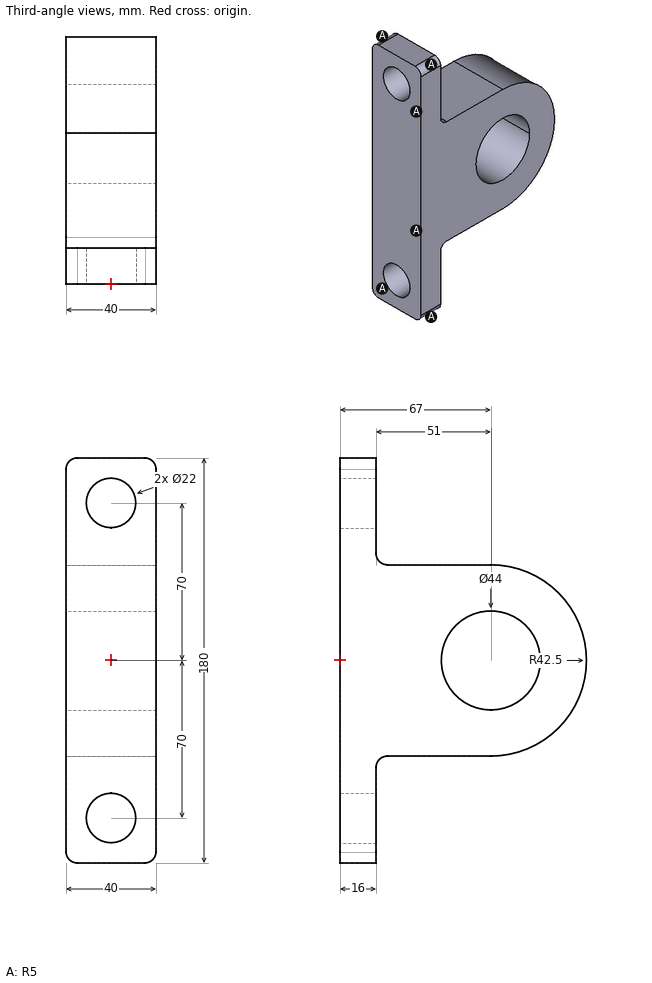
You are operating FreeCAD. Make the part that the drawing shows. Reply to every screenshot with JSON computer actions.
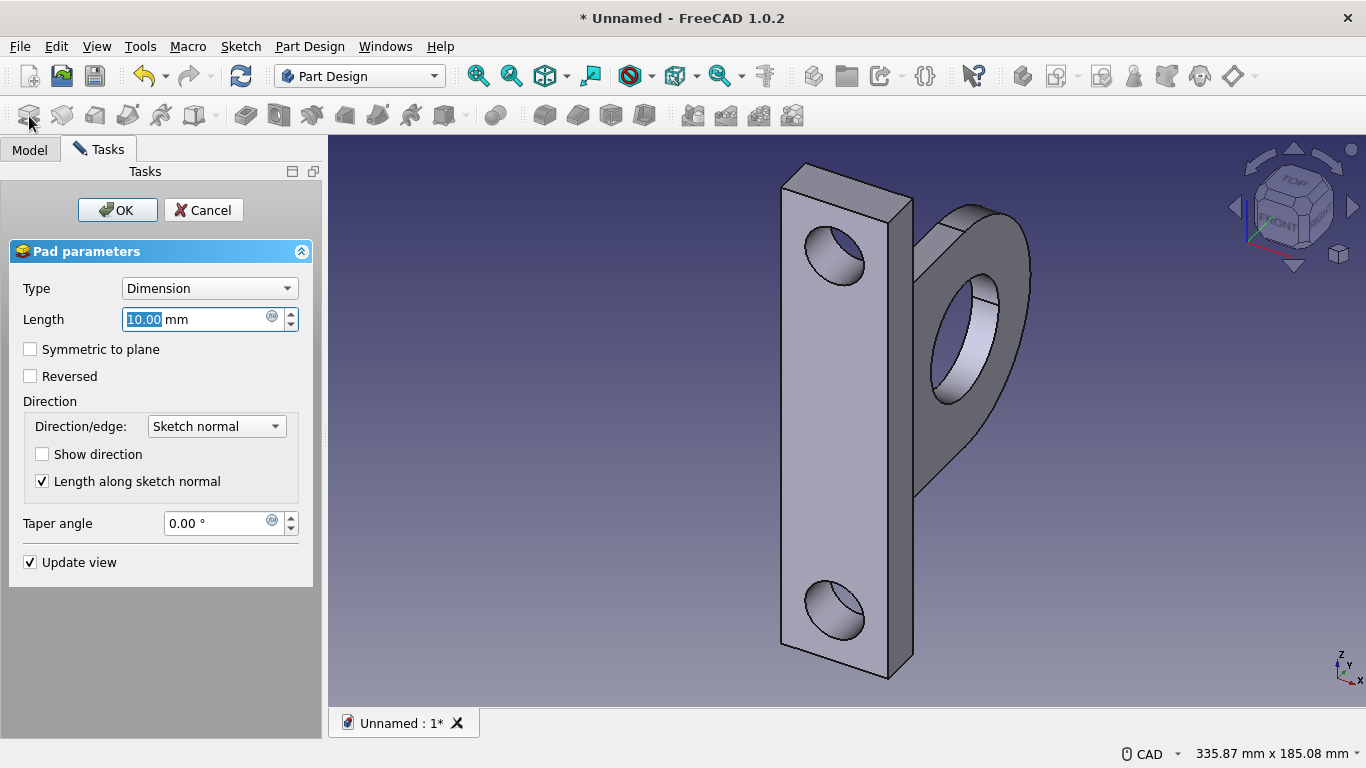
{"action": "type", "text": "40"}
{"action": "key", "text": "Tab"}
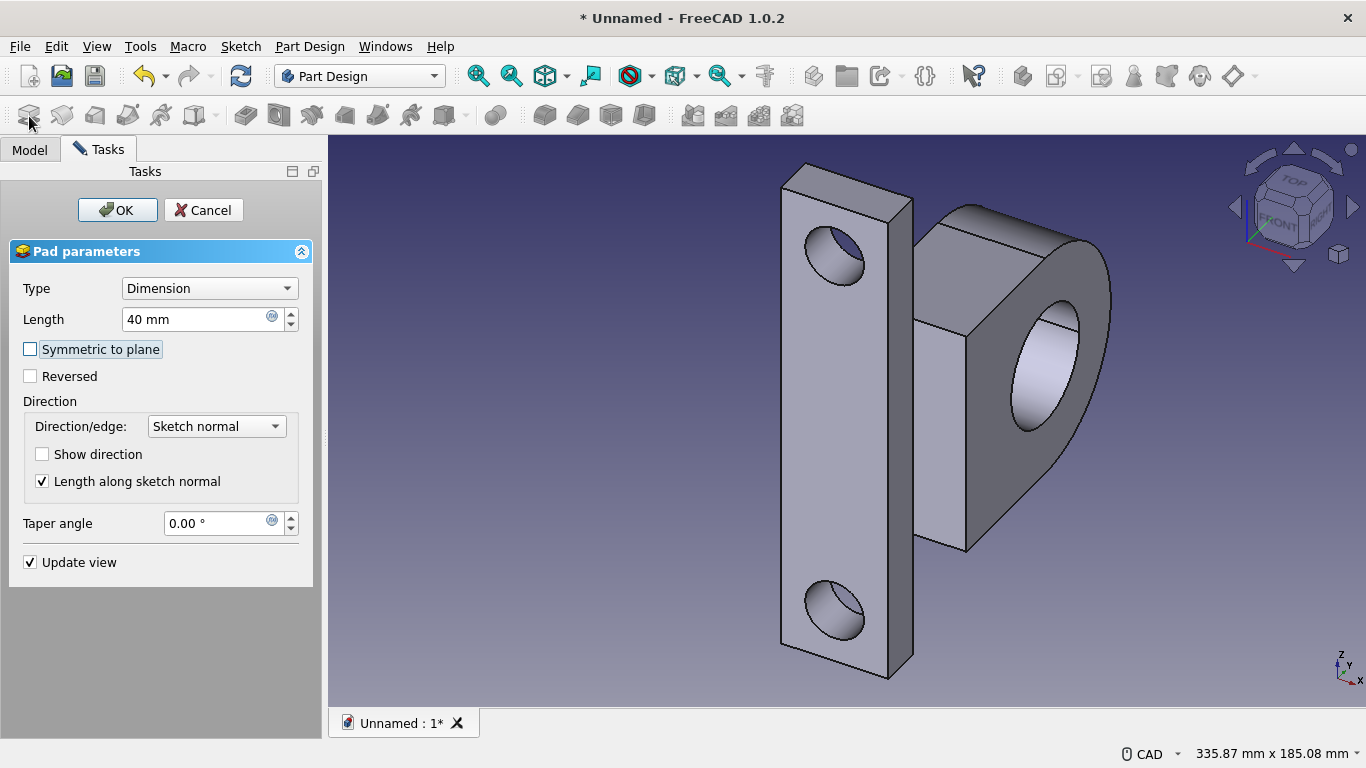
{"action": "left_click", "coordinate": [31, 349]}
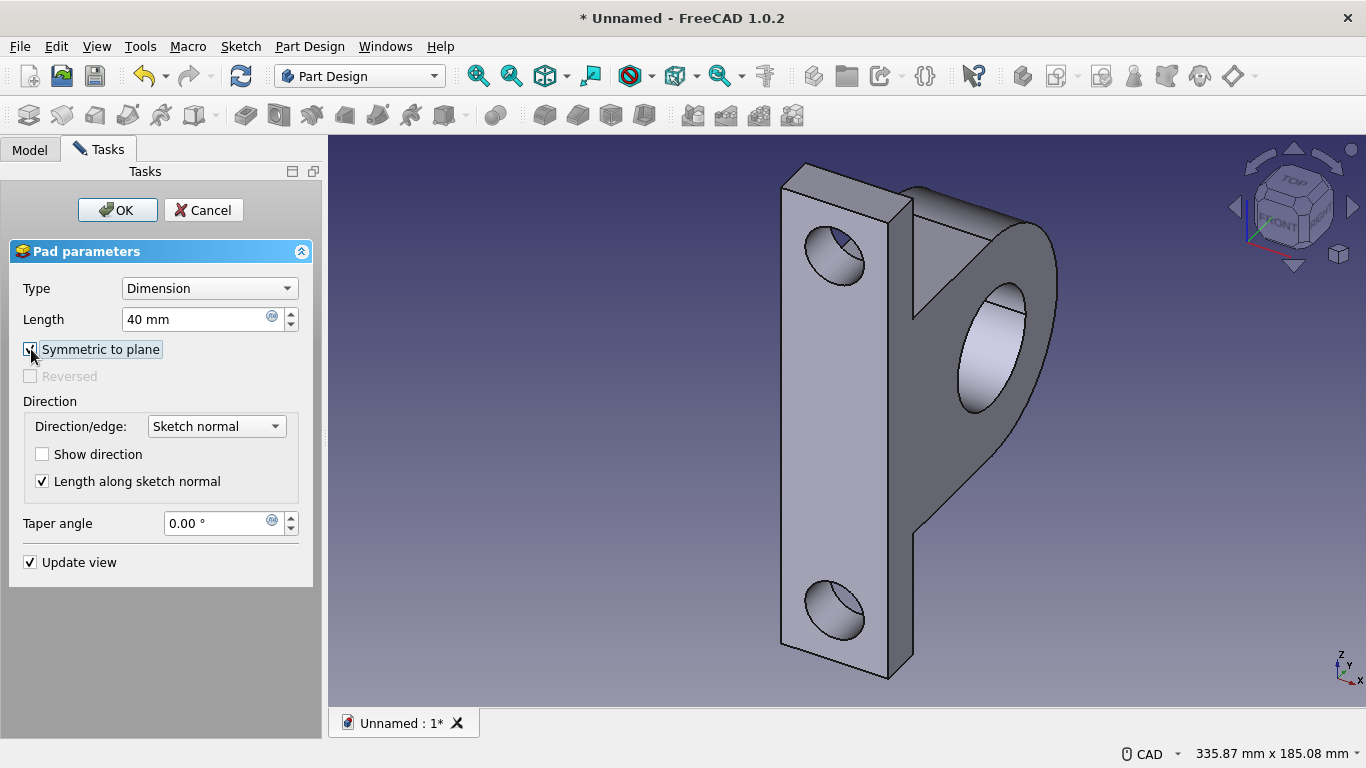
{"action": "left_click", "coordinate": [118, 210]}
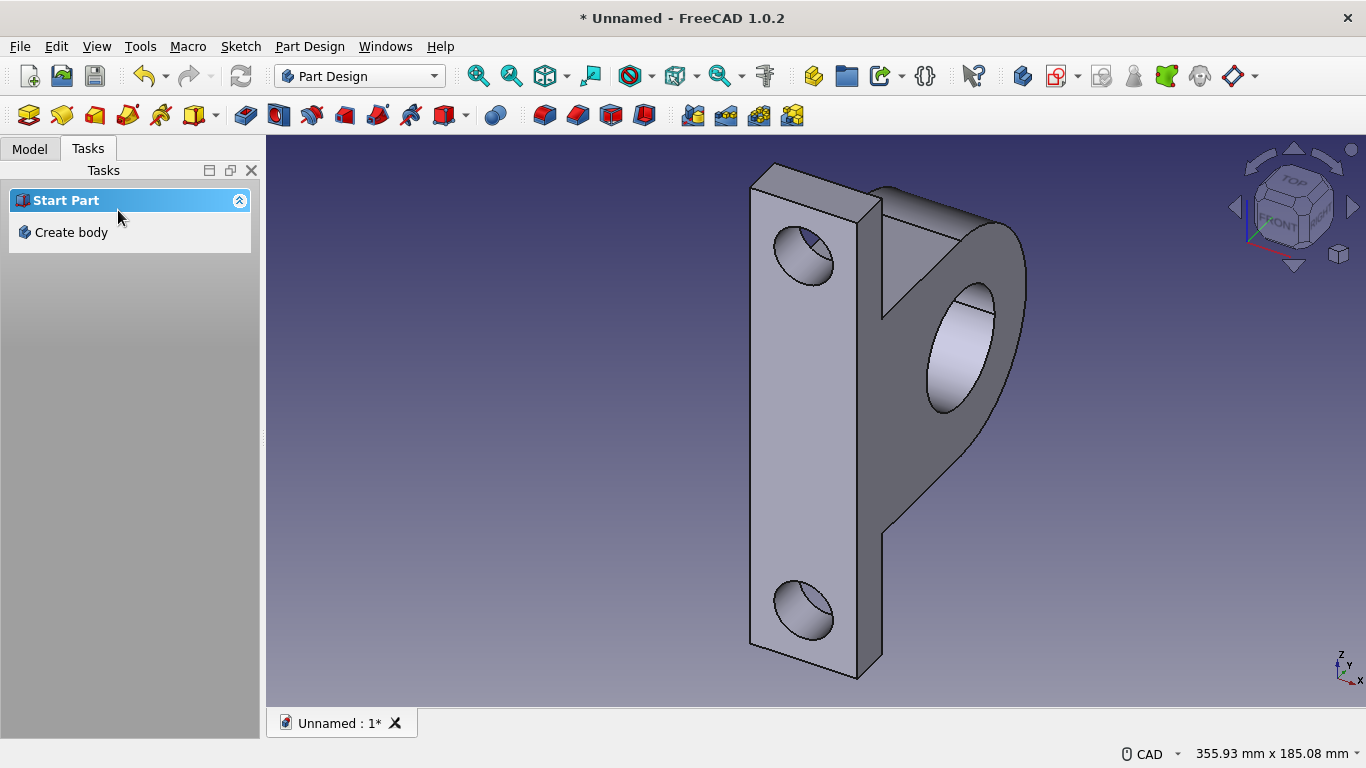
{"action": "key", "text": "v f"}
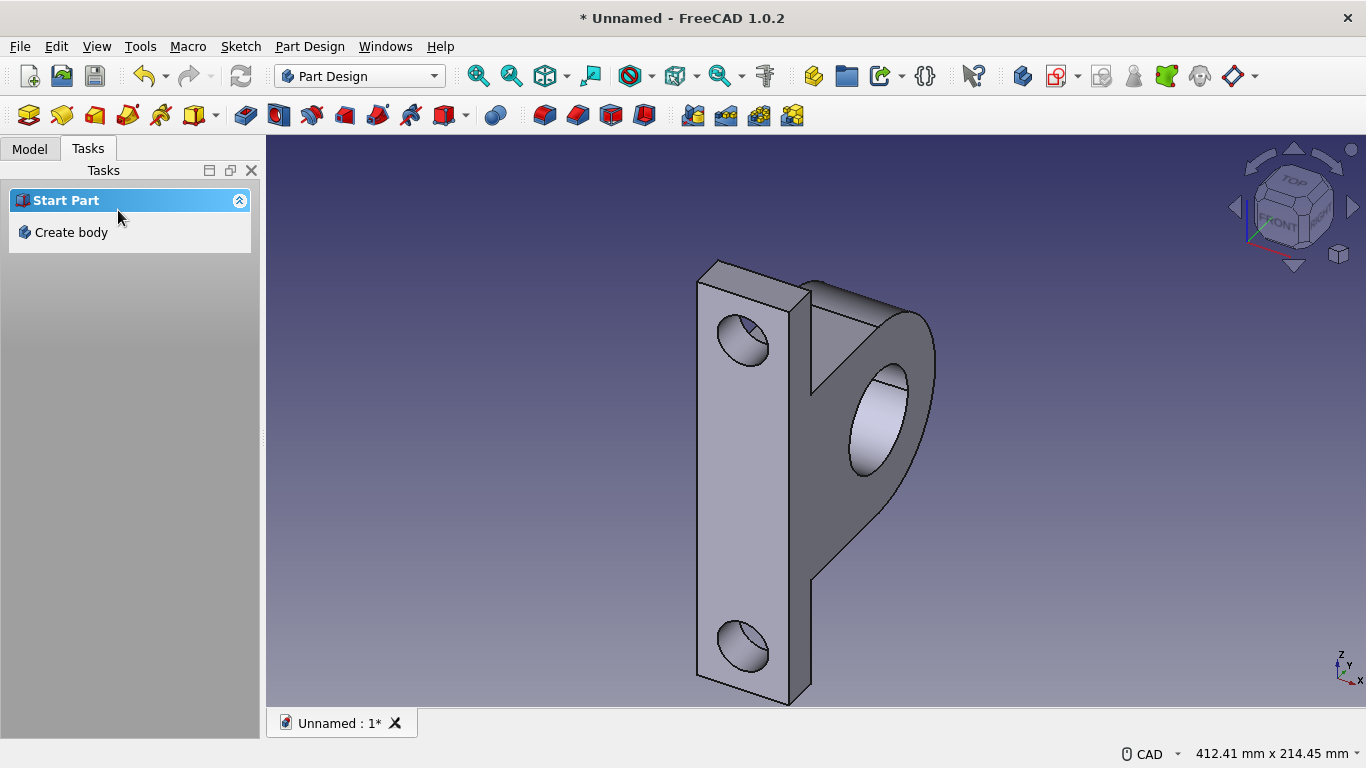
{"action": "left_click", "coordinate": [800, 301]}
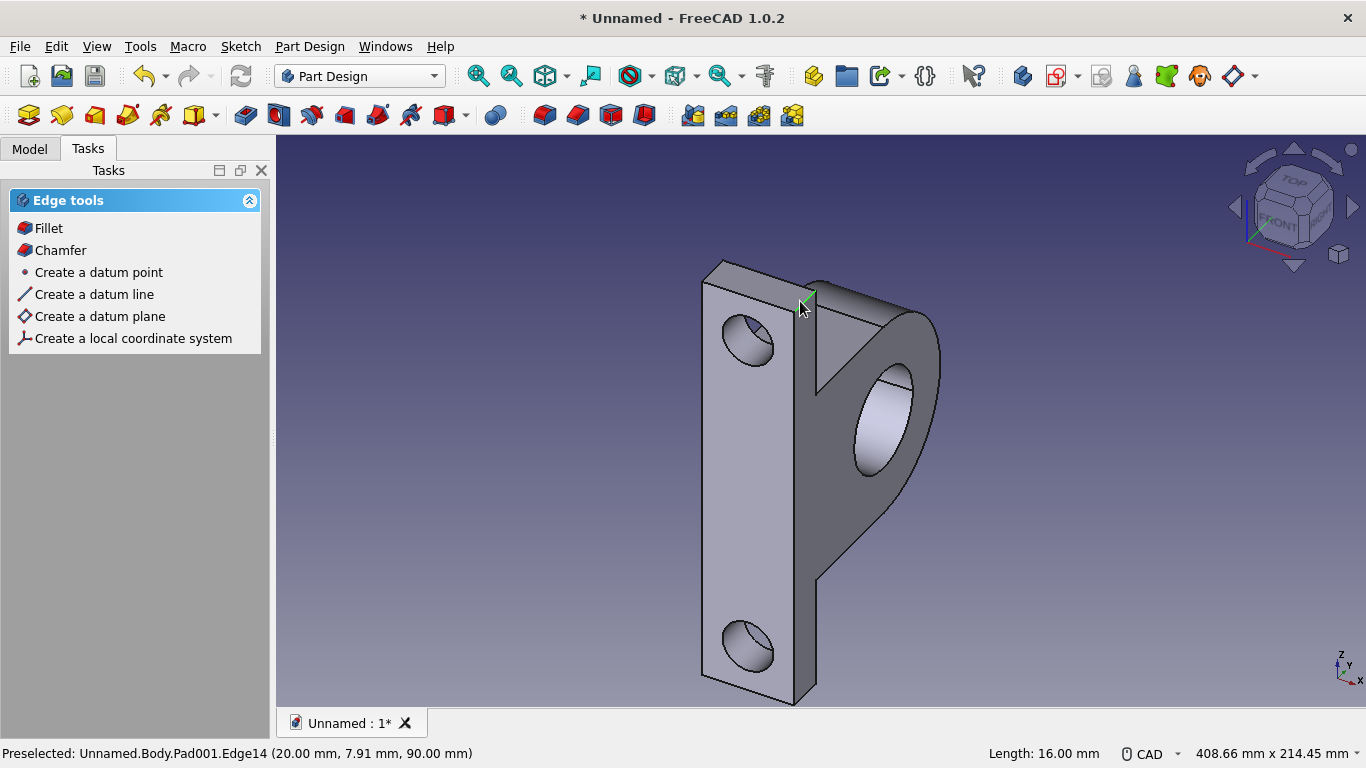
{"action": "key", "text": "0"}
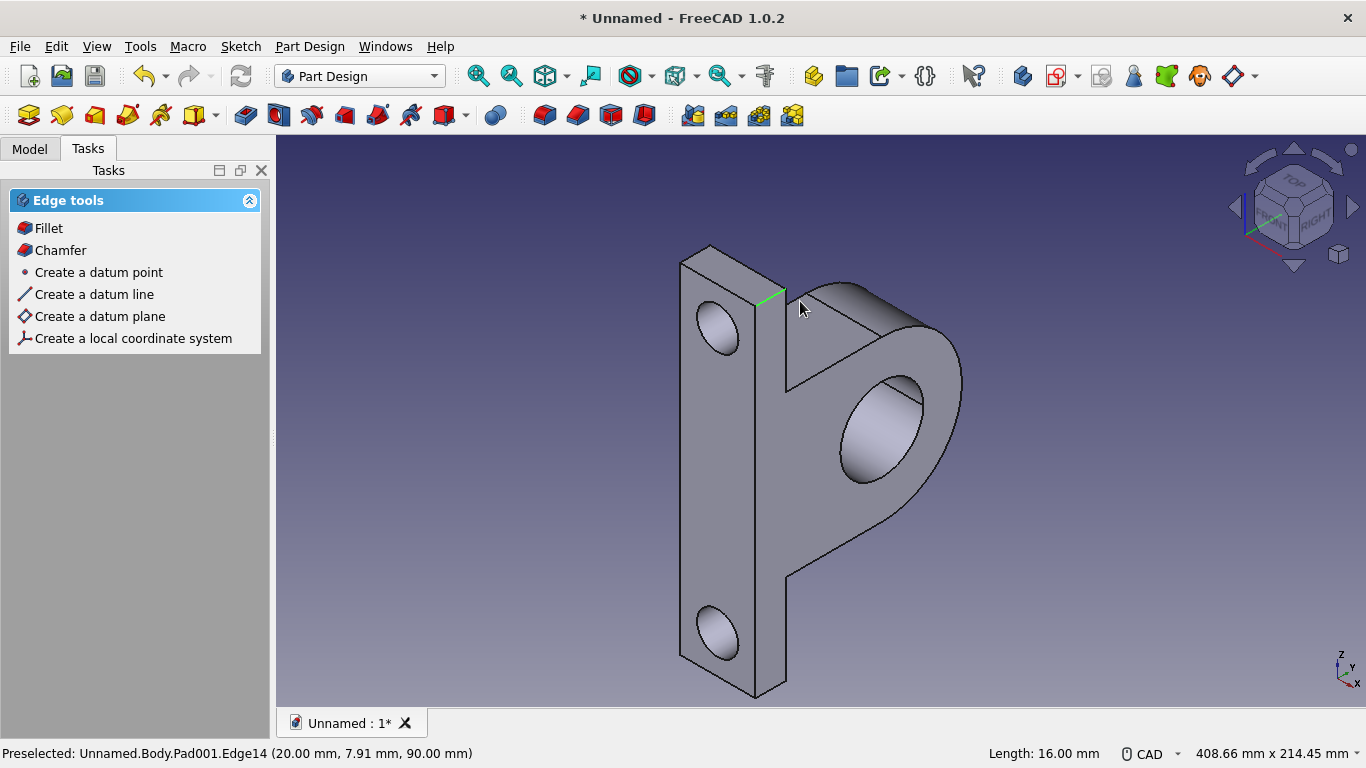
{"action": "key", "text": "2"}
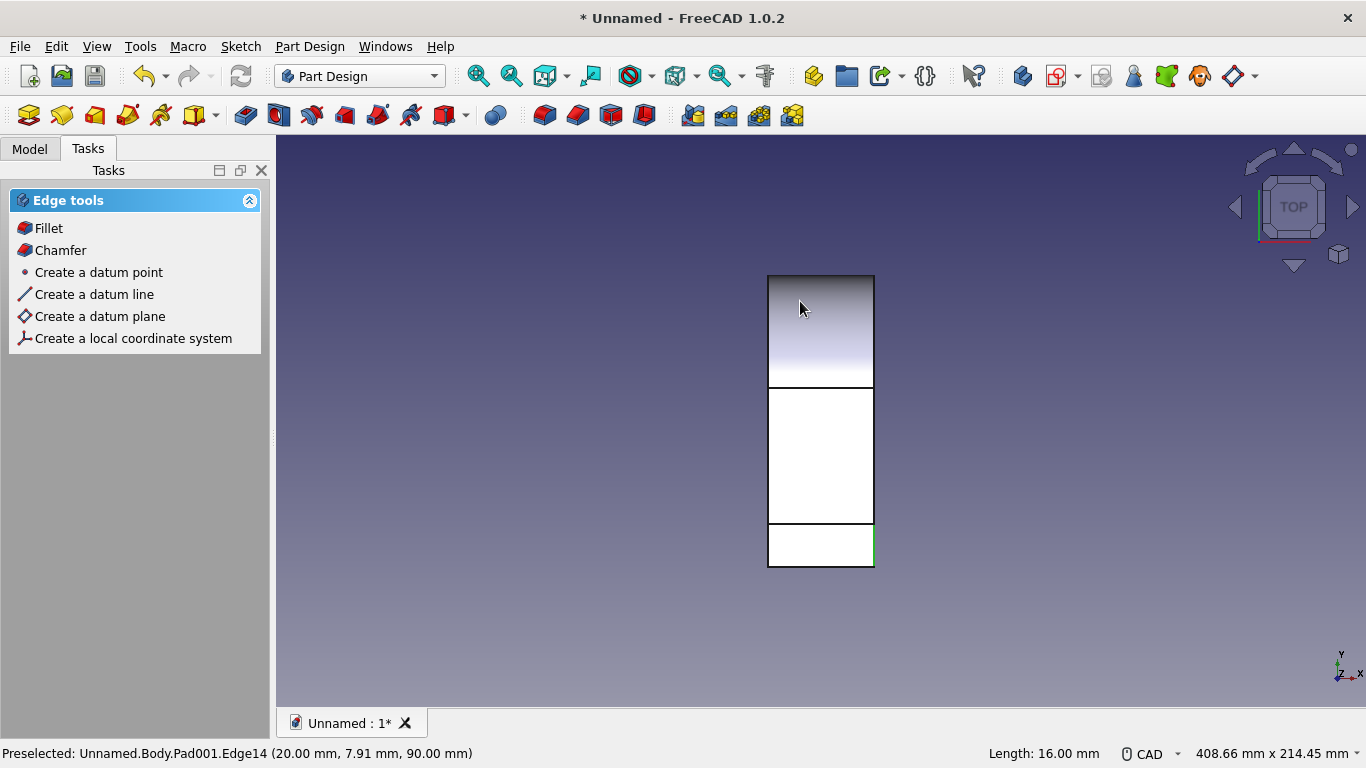
{"action": "left_click", "coordinate": [768, 545], "text": "ctrl"}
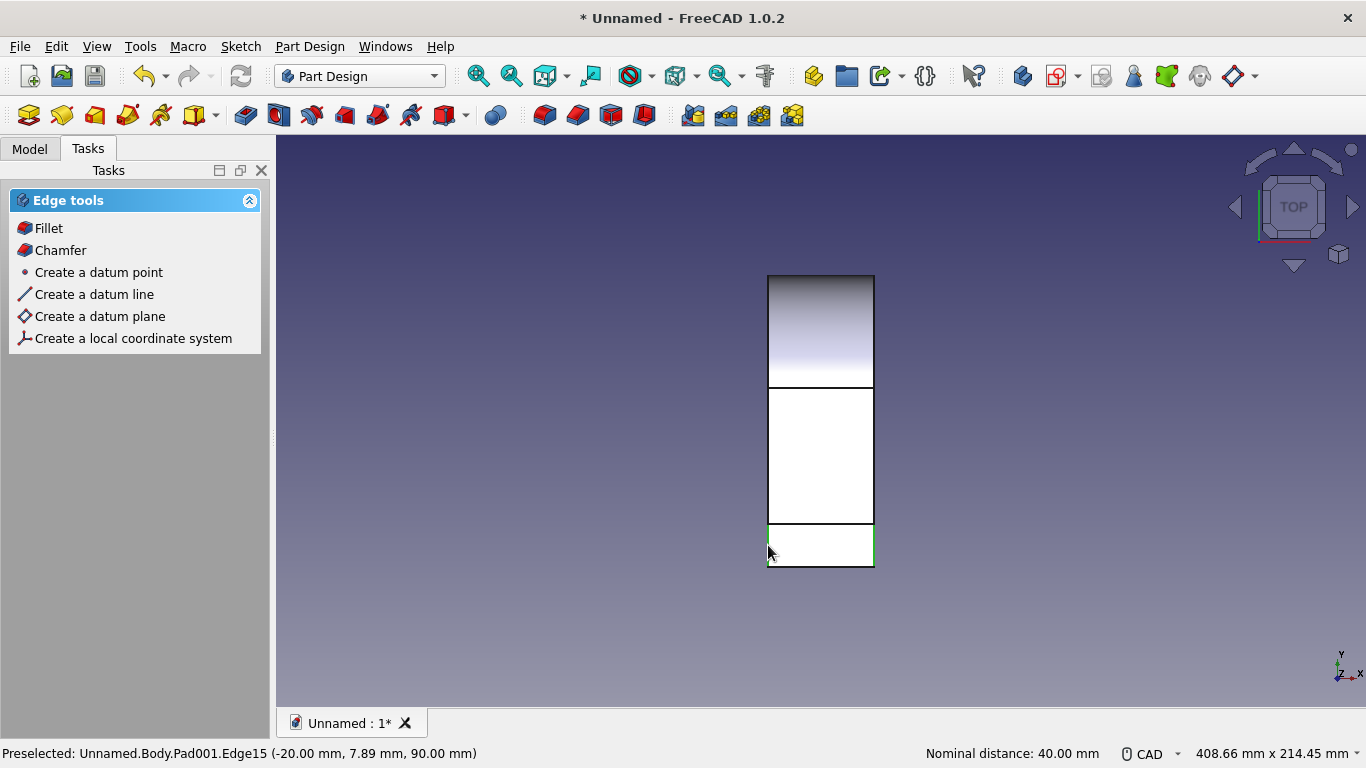
{"action": "key", "text": "1"}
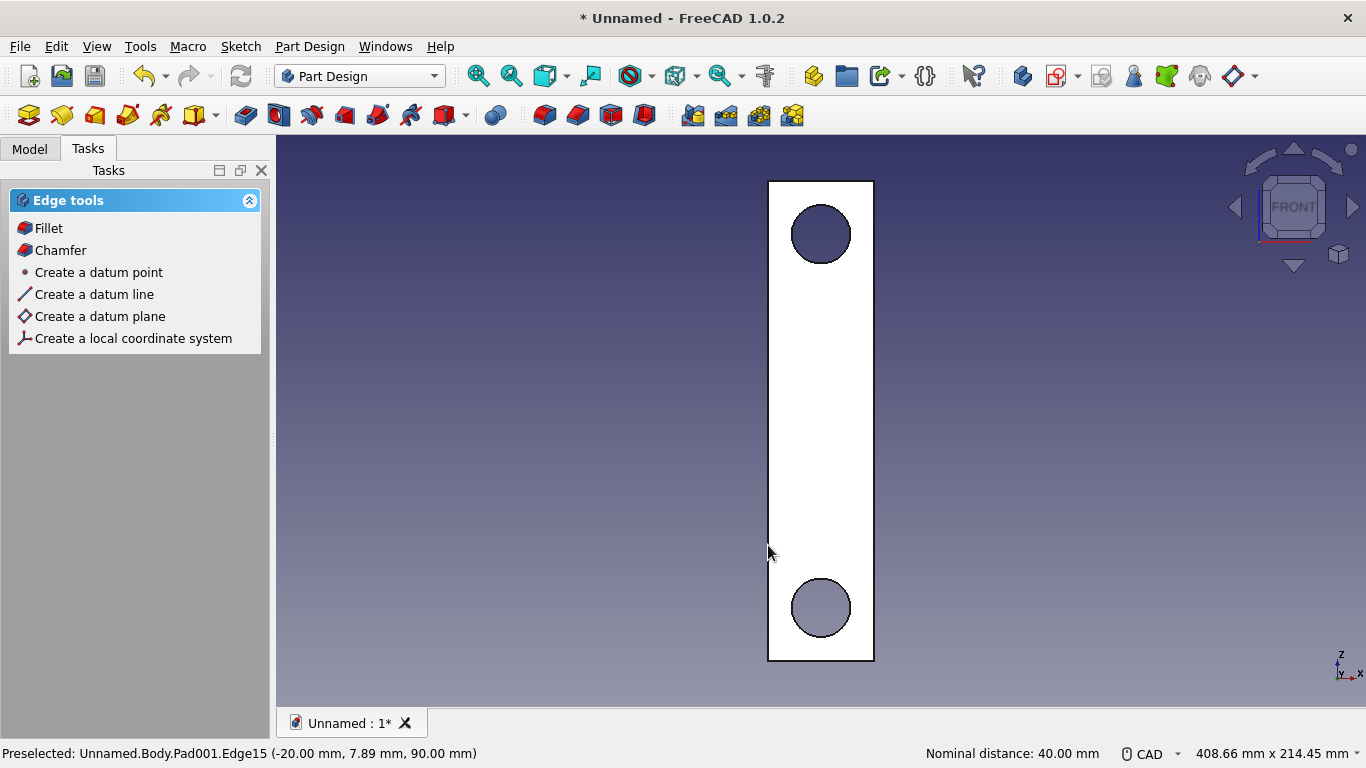
{"action": "key", "text": "3"}